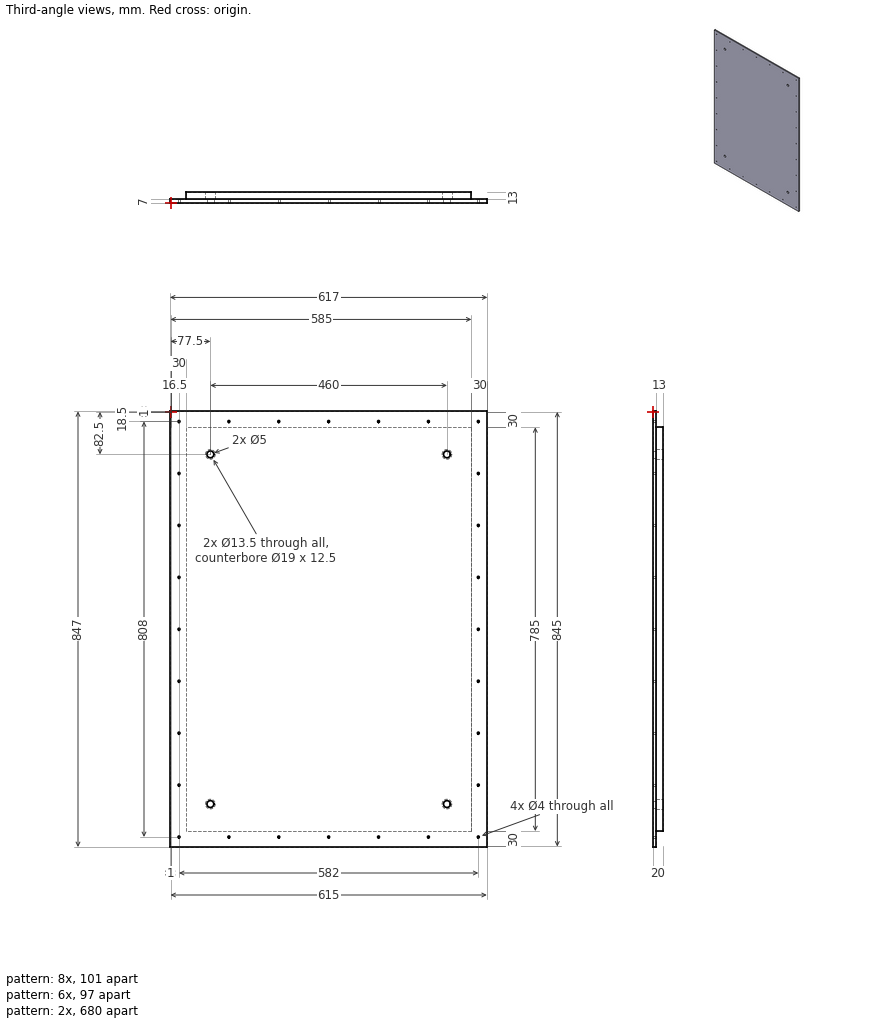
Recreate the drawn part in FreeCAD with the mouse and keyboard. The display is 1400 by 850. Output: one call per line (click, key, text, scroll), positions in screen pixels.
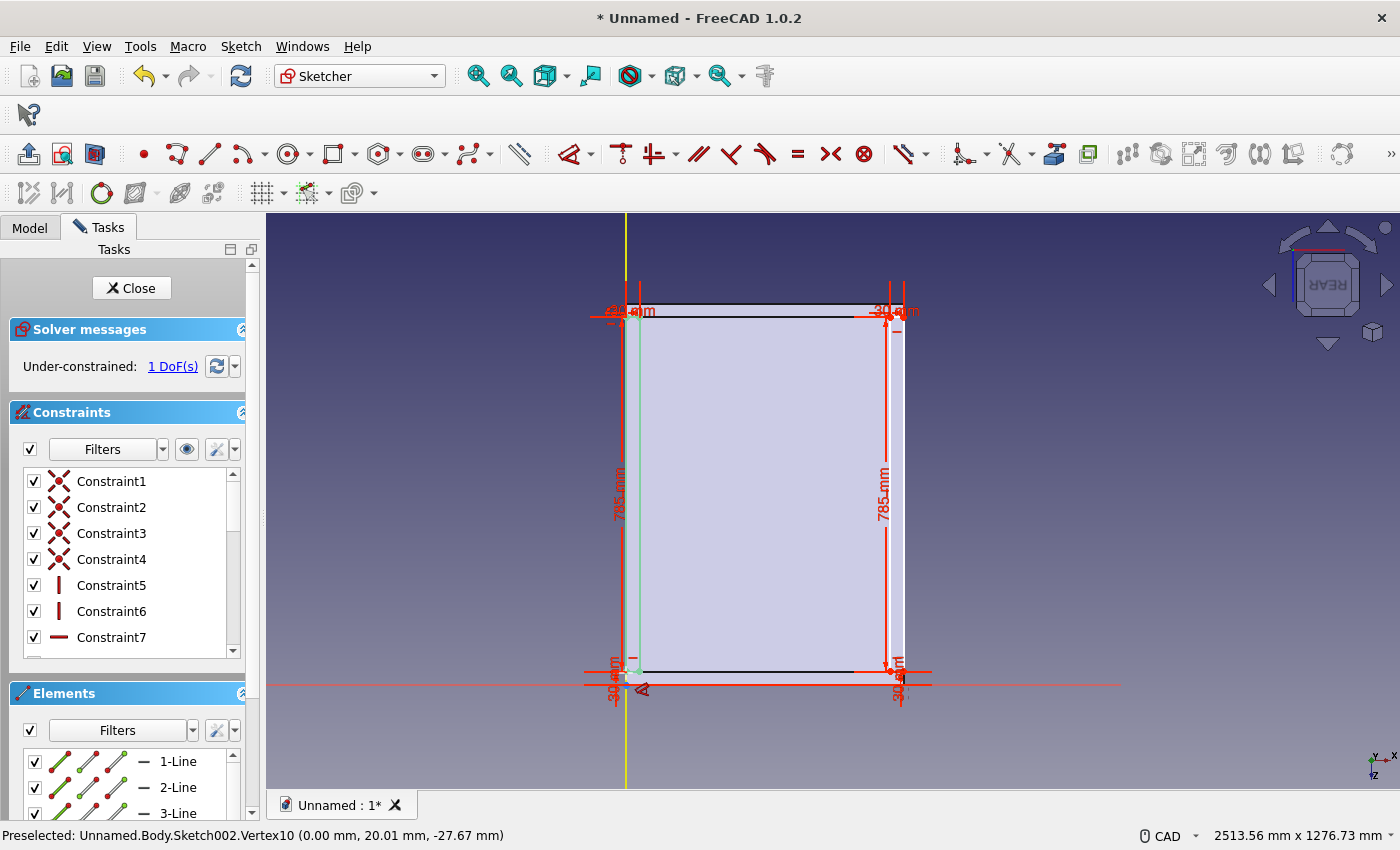
click(890, 317)
click(758, 719)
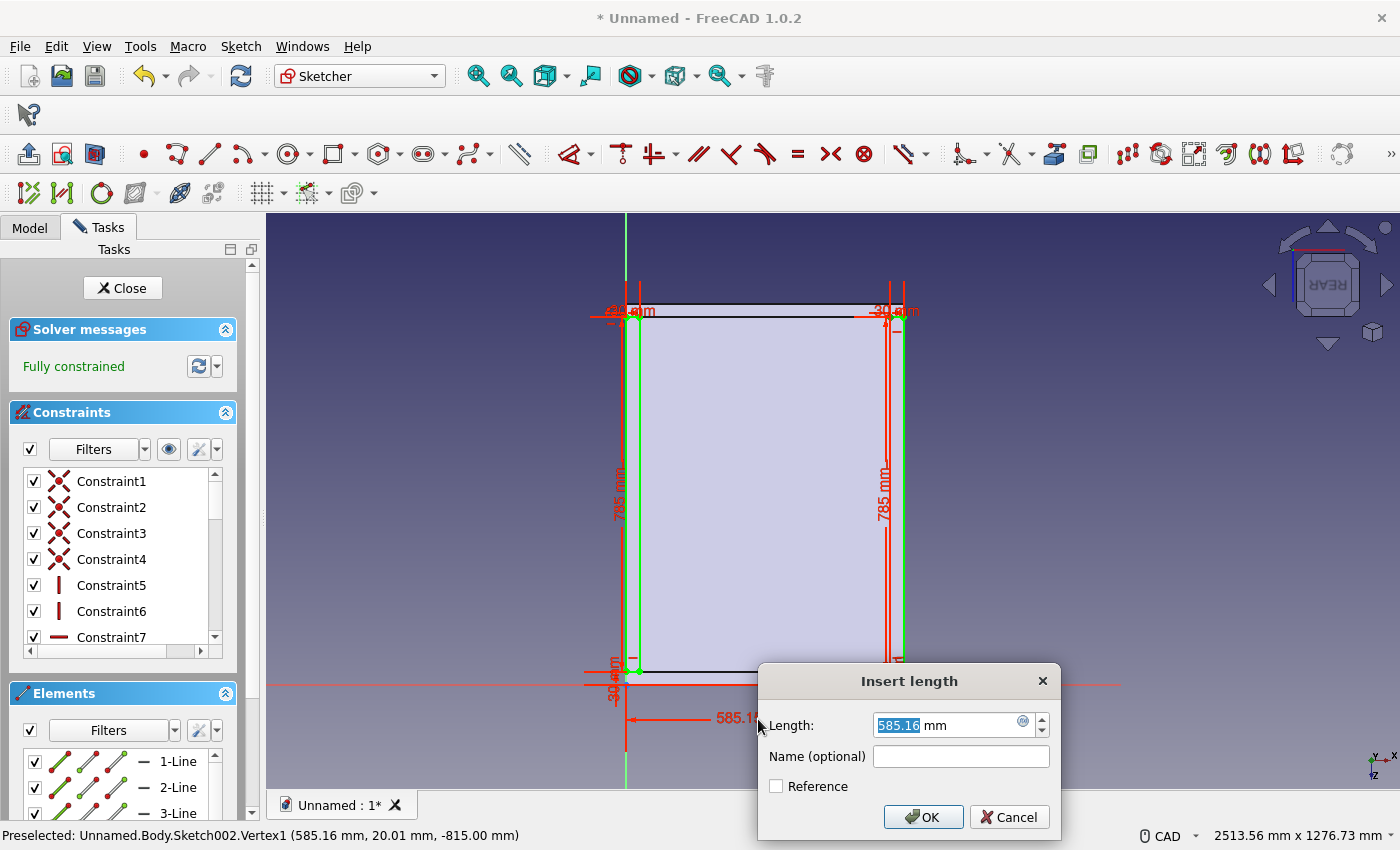
text(585)
key(Return)
key(Escape)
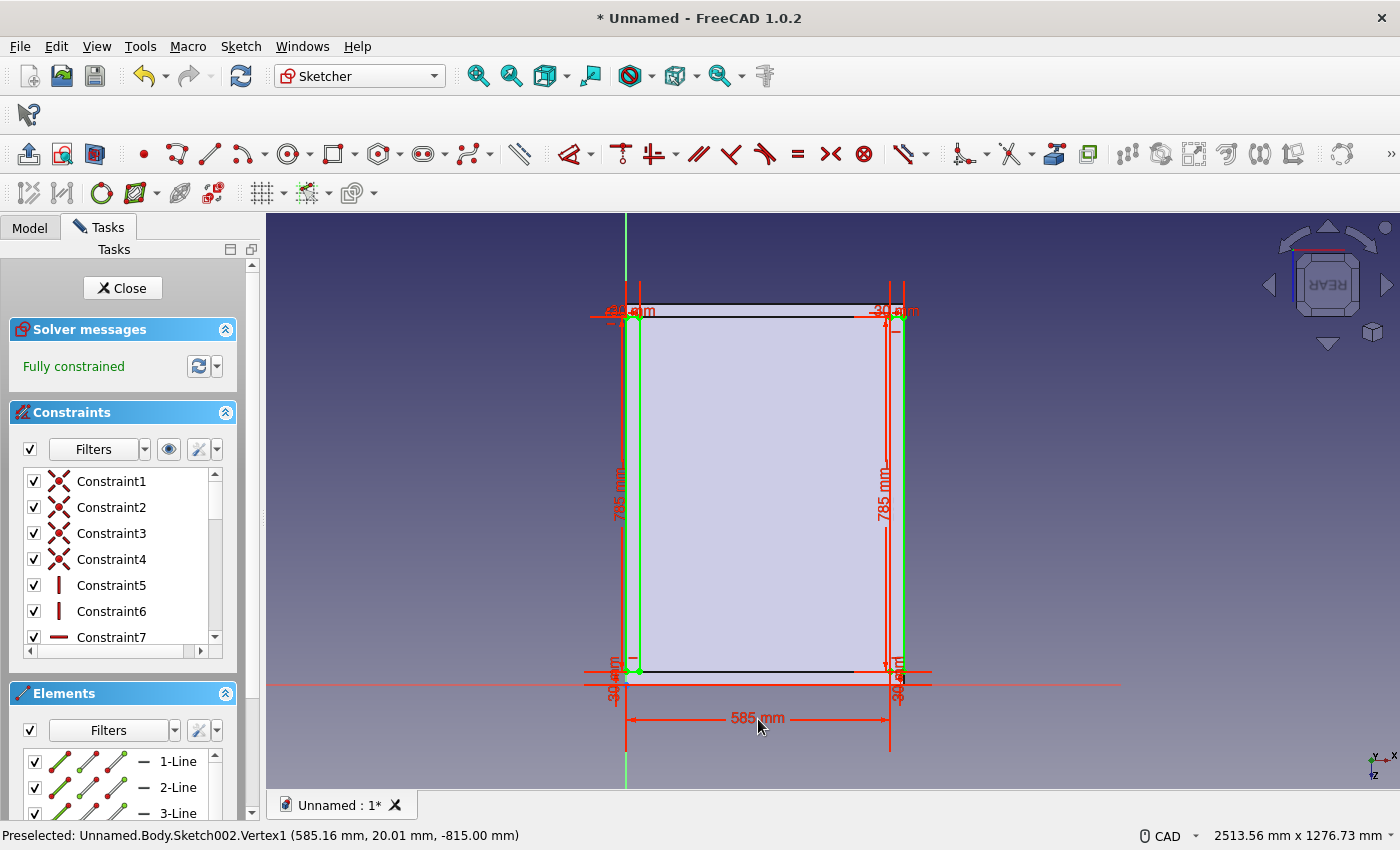
click(123, 288)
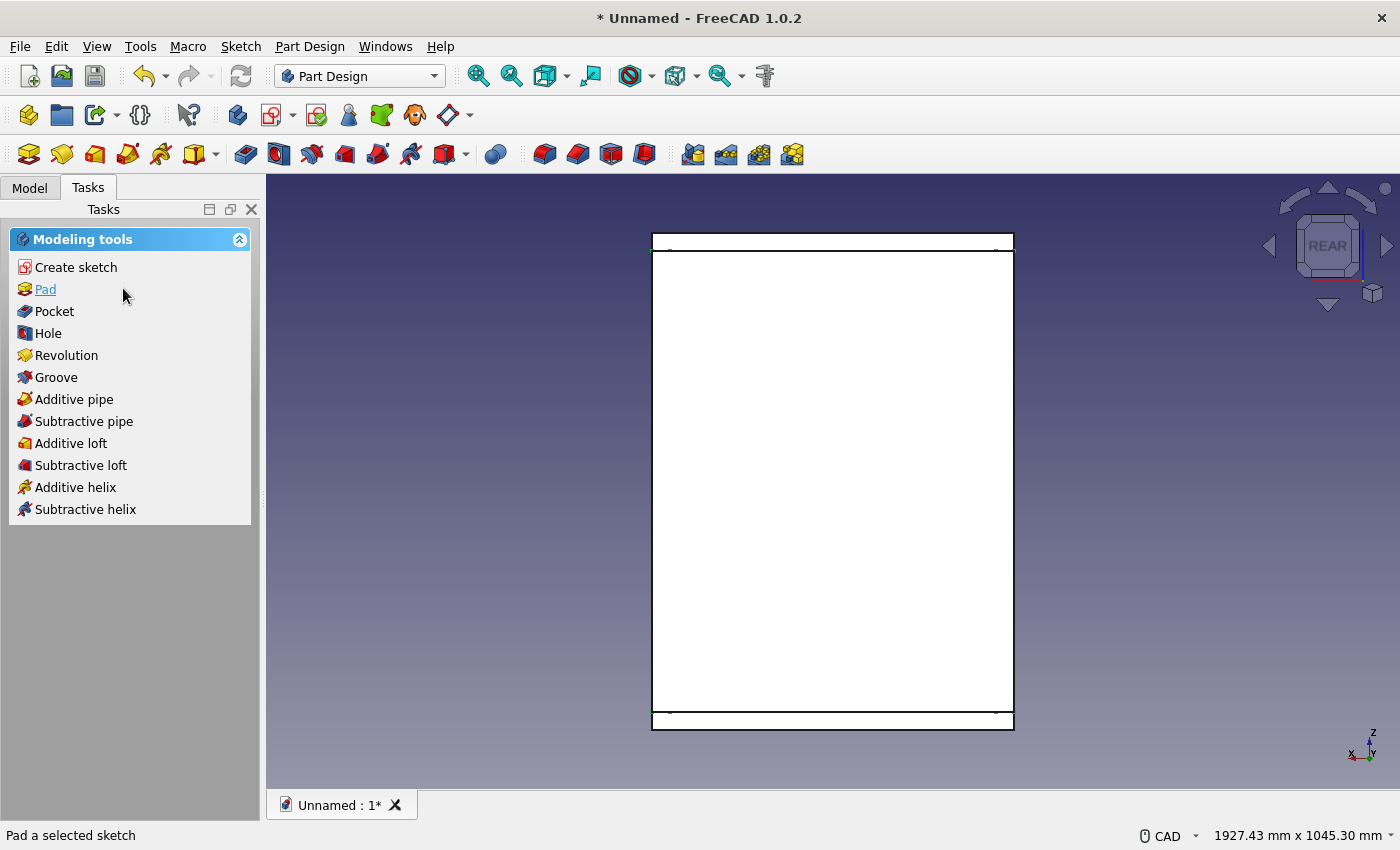
click(246, 154)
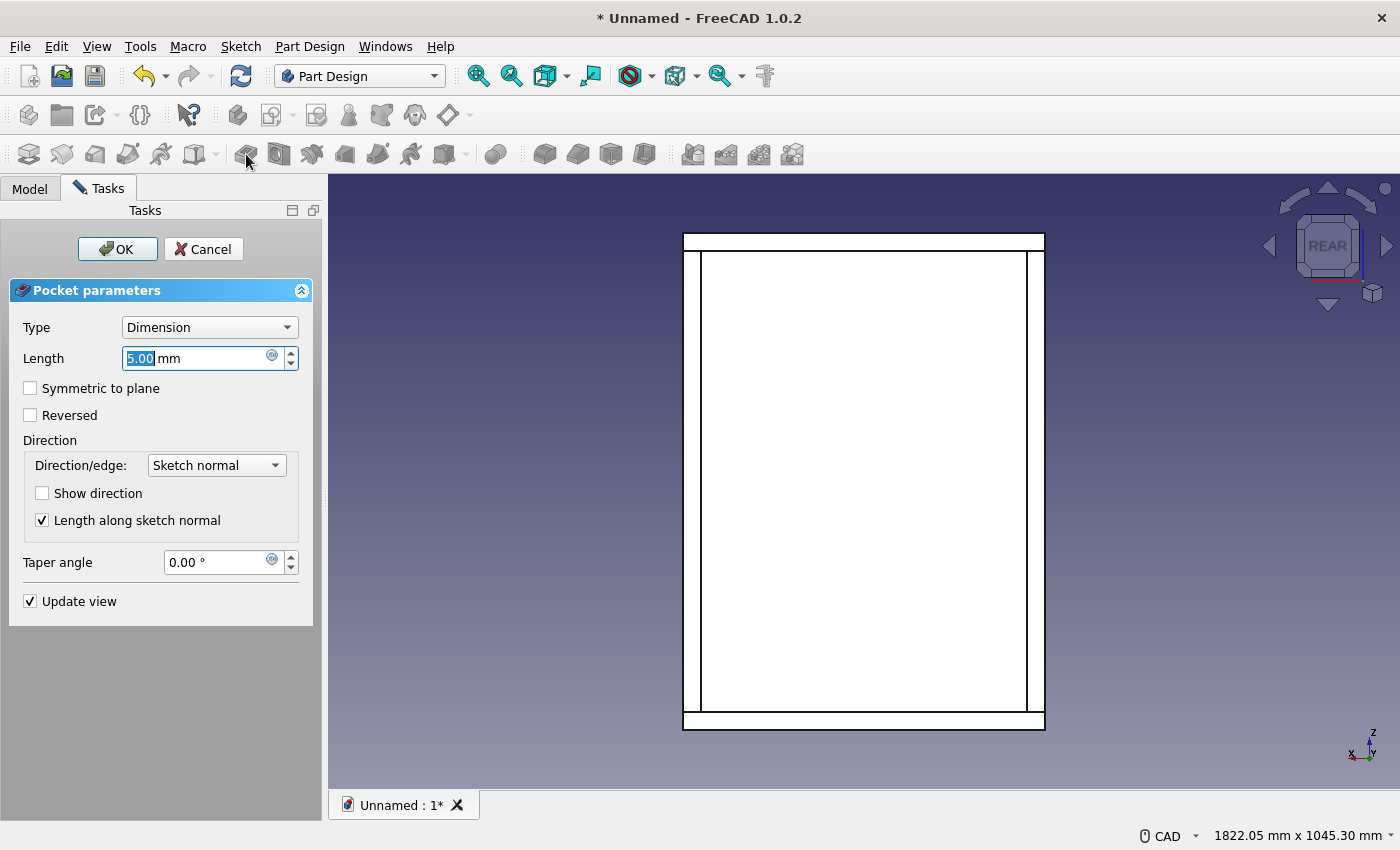
text(13)
key(Tab)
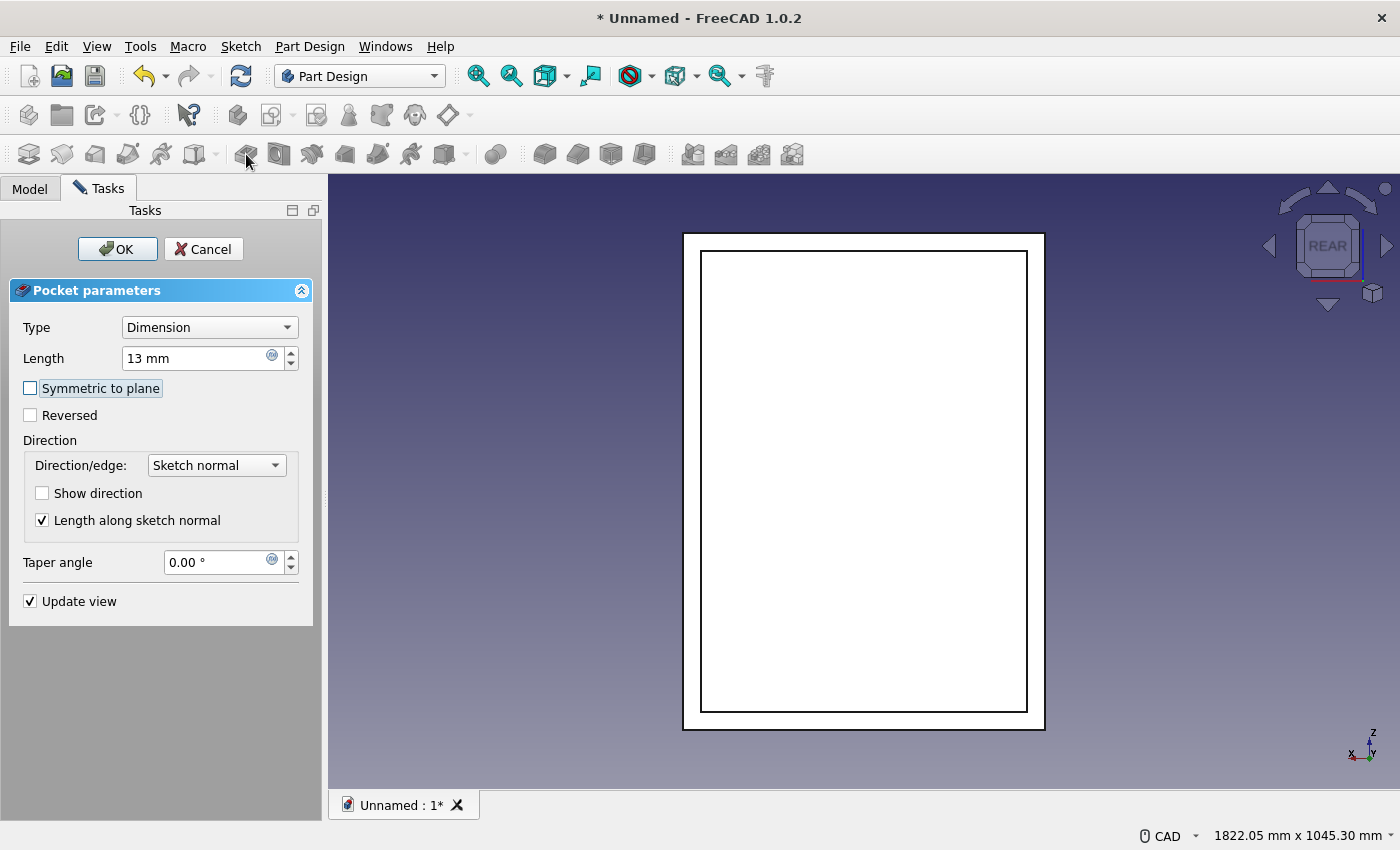
click(118, 249)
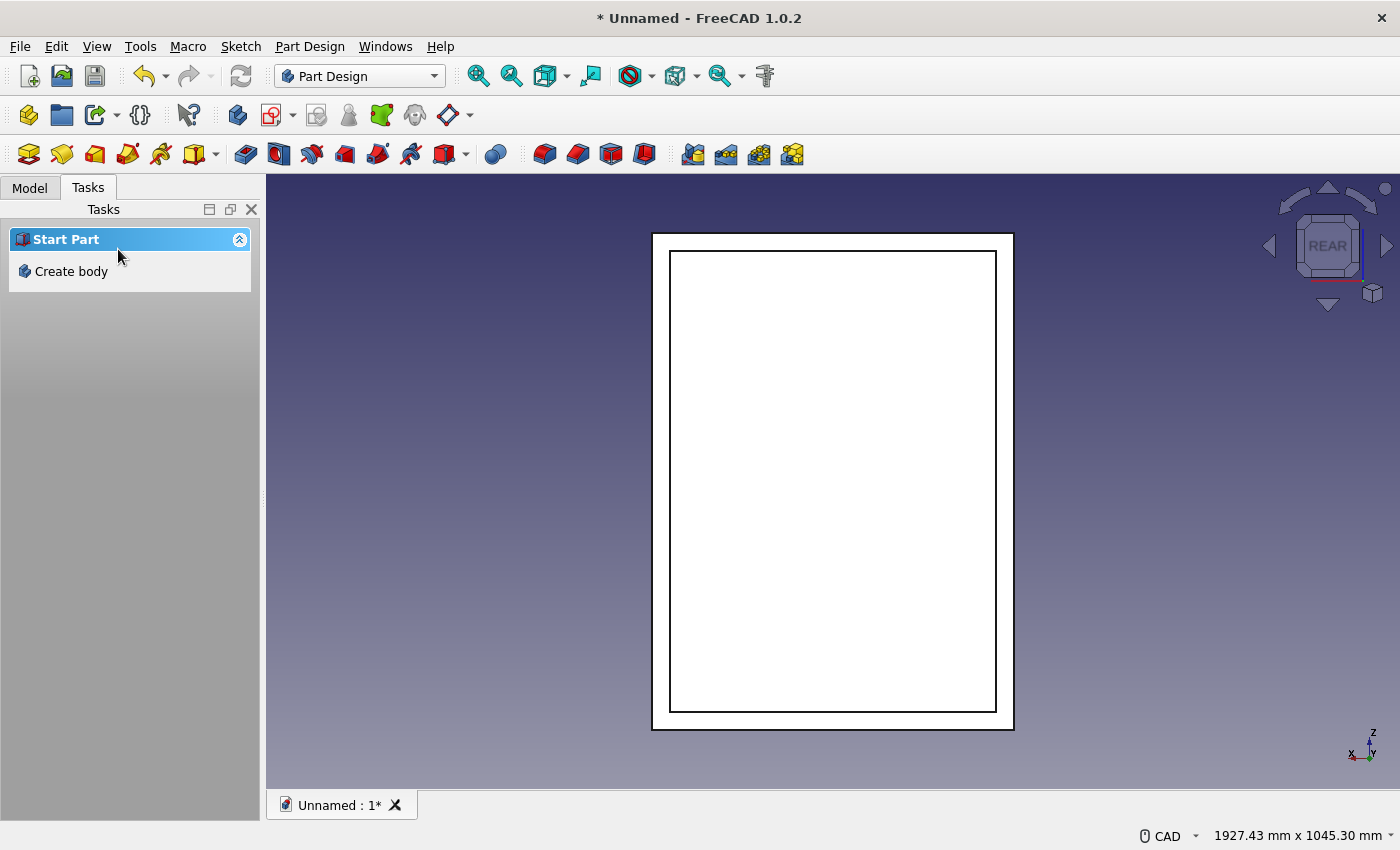
click(658, 557)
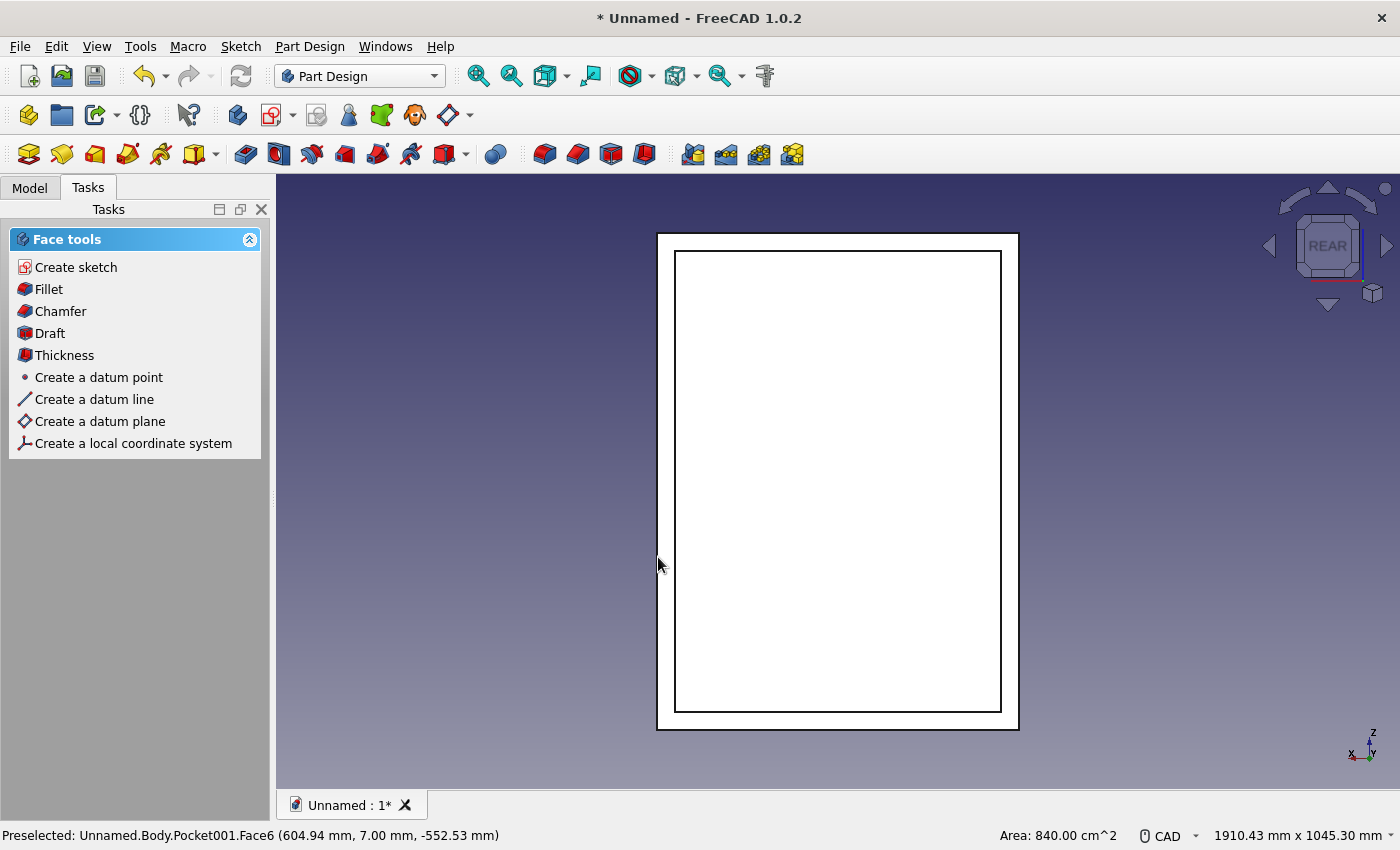
click(270, 116)